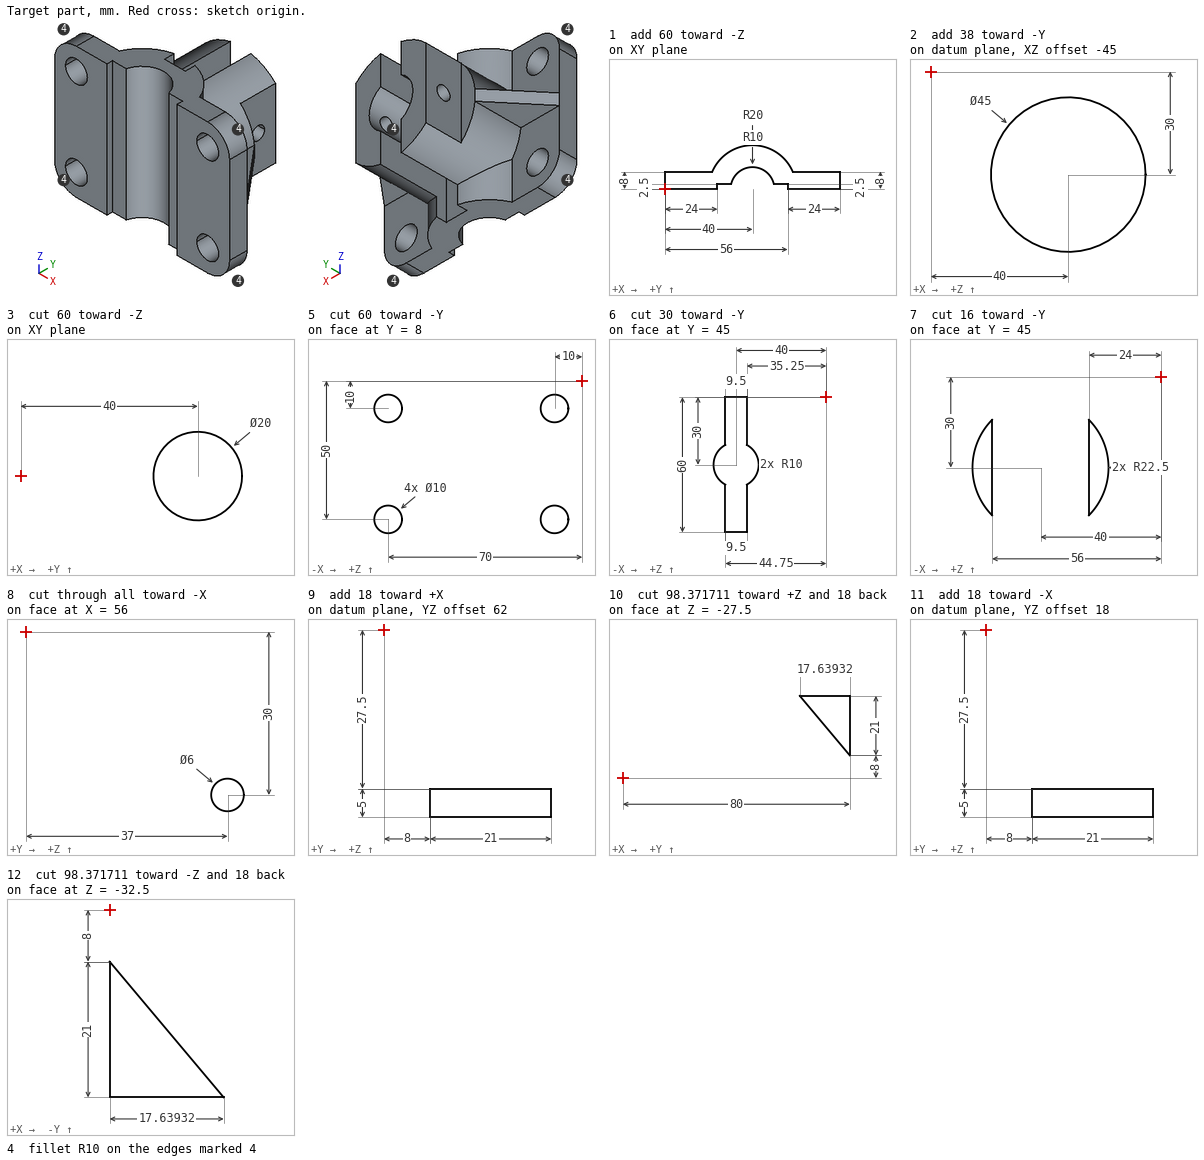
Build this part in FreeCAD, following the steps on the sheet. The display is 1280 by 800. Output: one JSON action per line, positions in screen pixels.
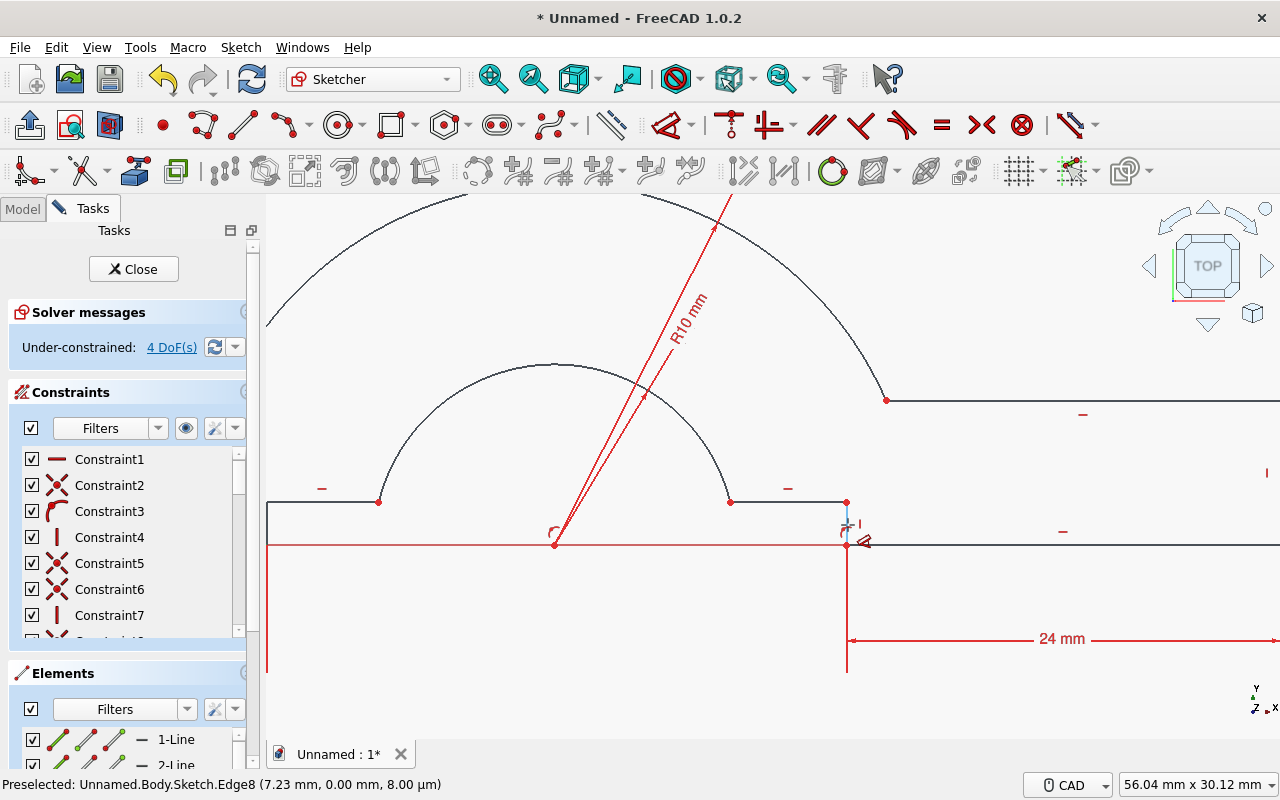
{"action": "left_click", "coordinate": [847, 524]}
{"action": "left_click", "coordinate": [881, 524]}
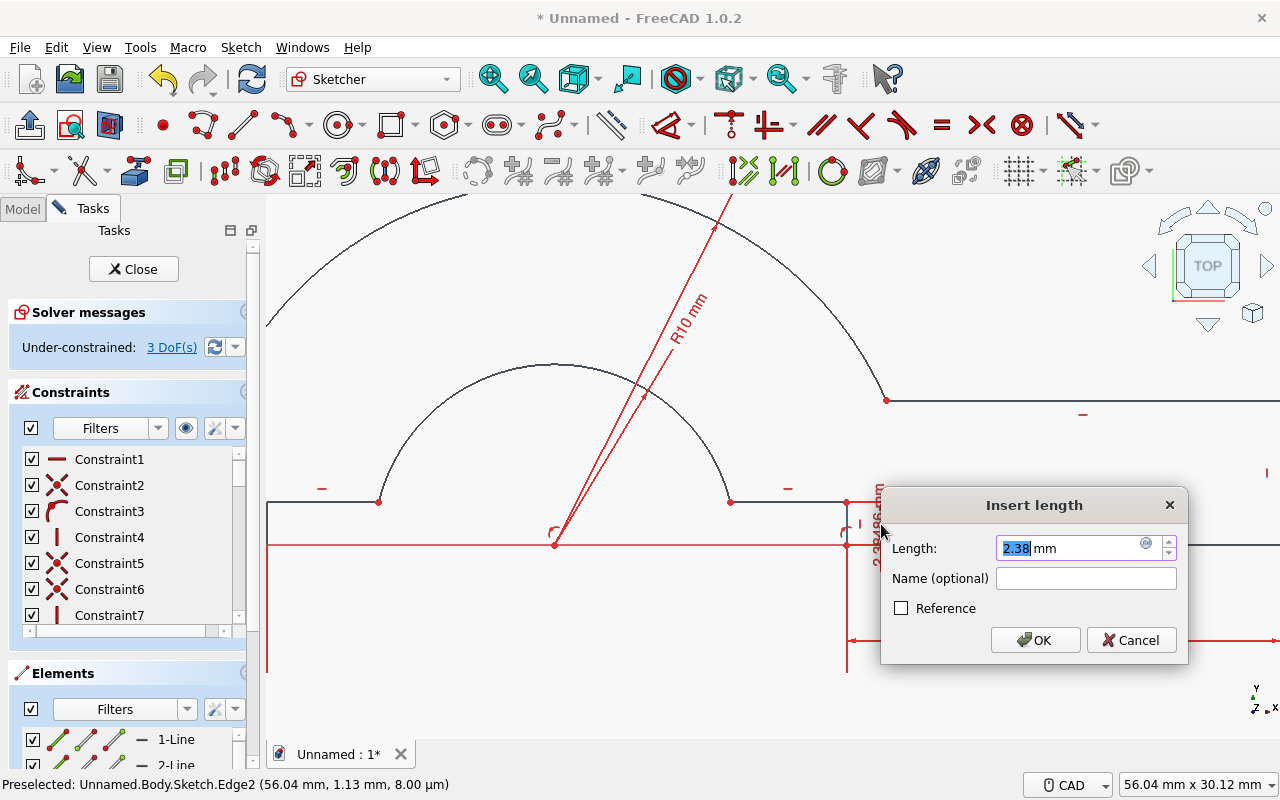
{"action": "type", "text": "2.5"}
{"action": "key", "text": "Return"}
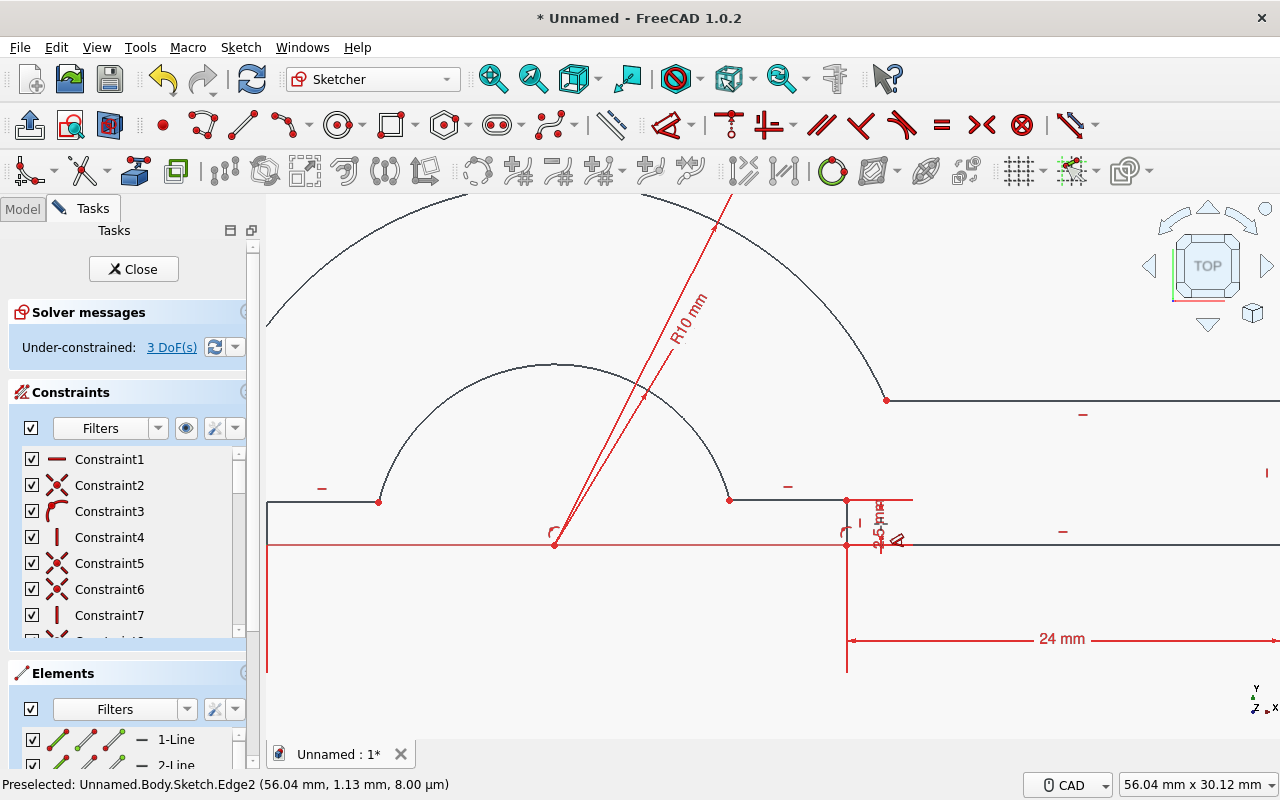
{"action": "scroll", "coordinate": [791, 526], "scroll_direction": "down", "scroll_amount": 5}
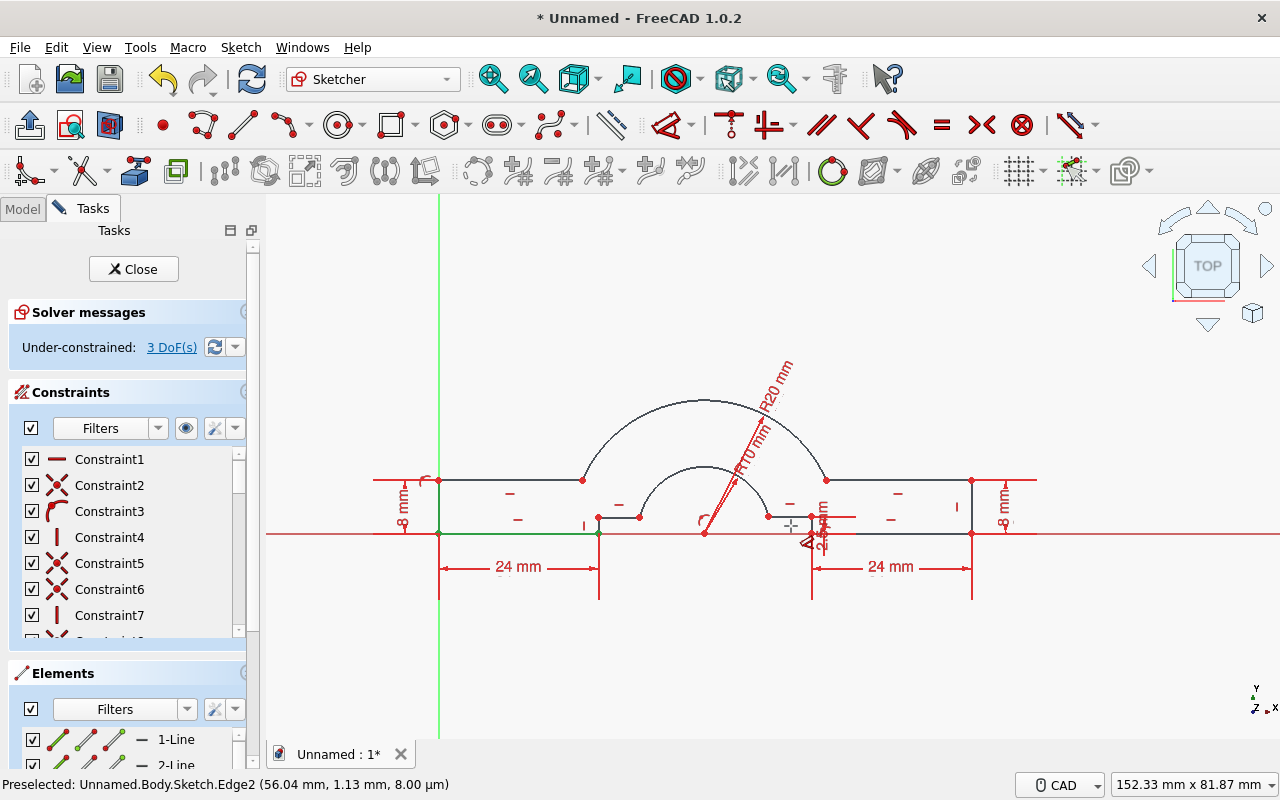
{"action": "scroll", "coordinate": [599, 529], "scroll_direction": "up", "scroll_amount": 6}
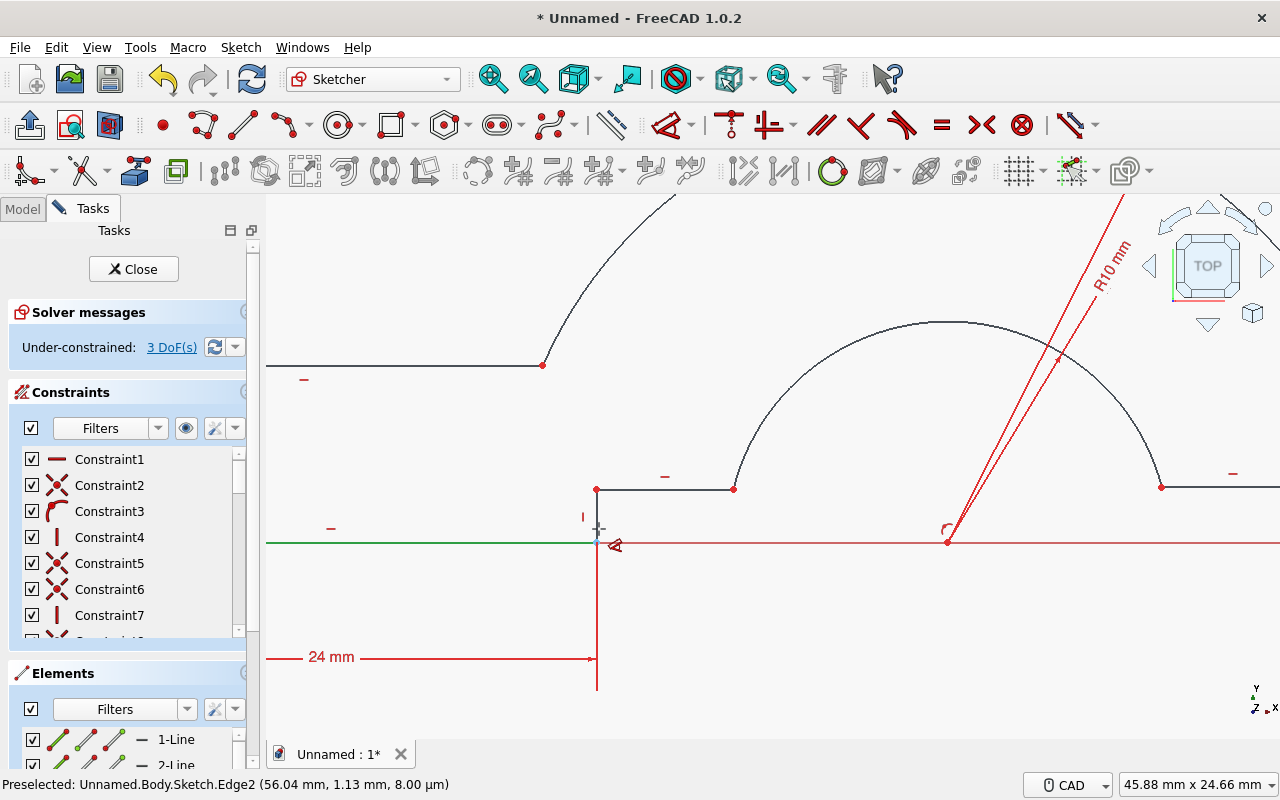
{"action": "left_click", "coordinate": [597, 527]}
{"action": "left_click", "coordinate": [563, 516]}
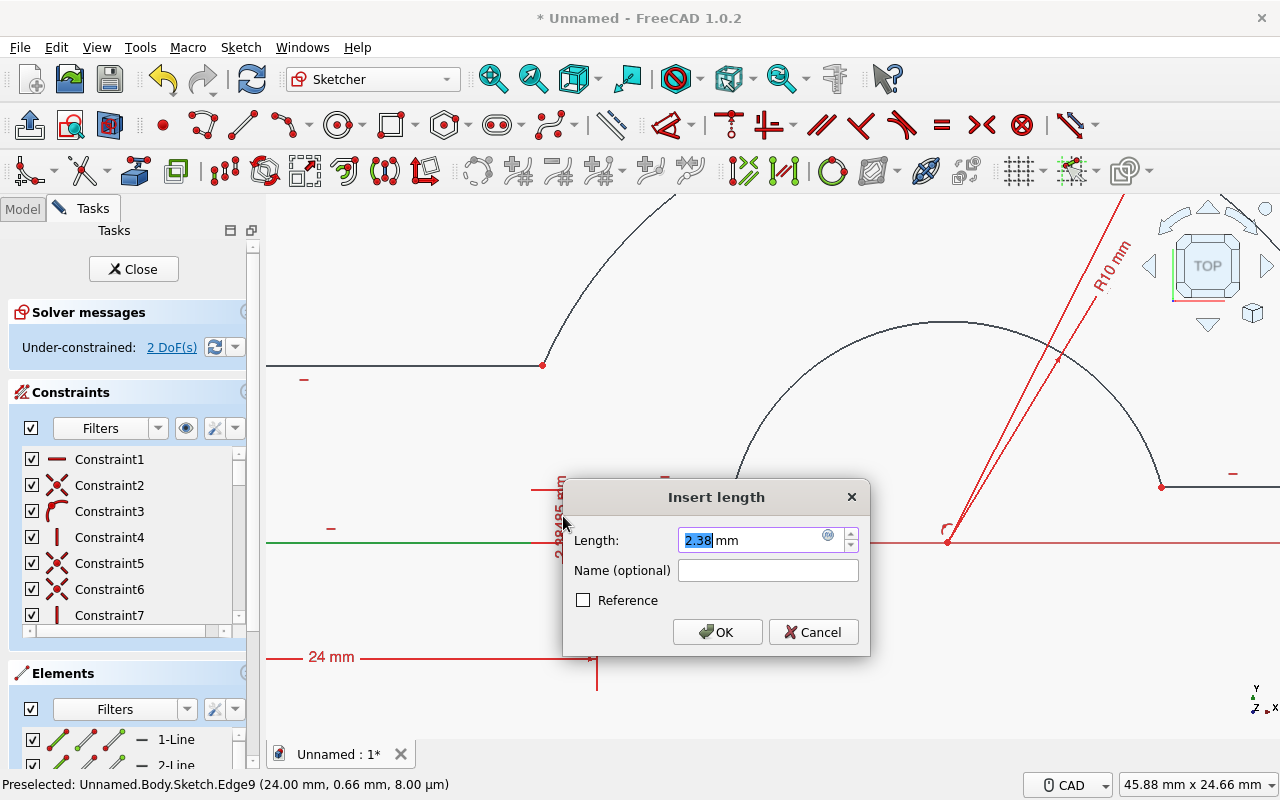
{"action": "type", "text": "2.5"}
{"action": "key", "text": "Return"}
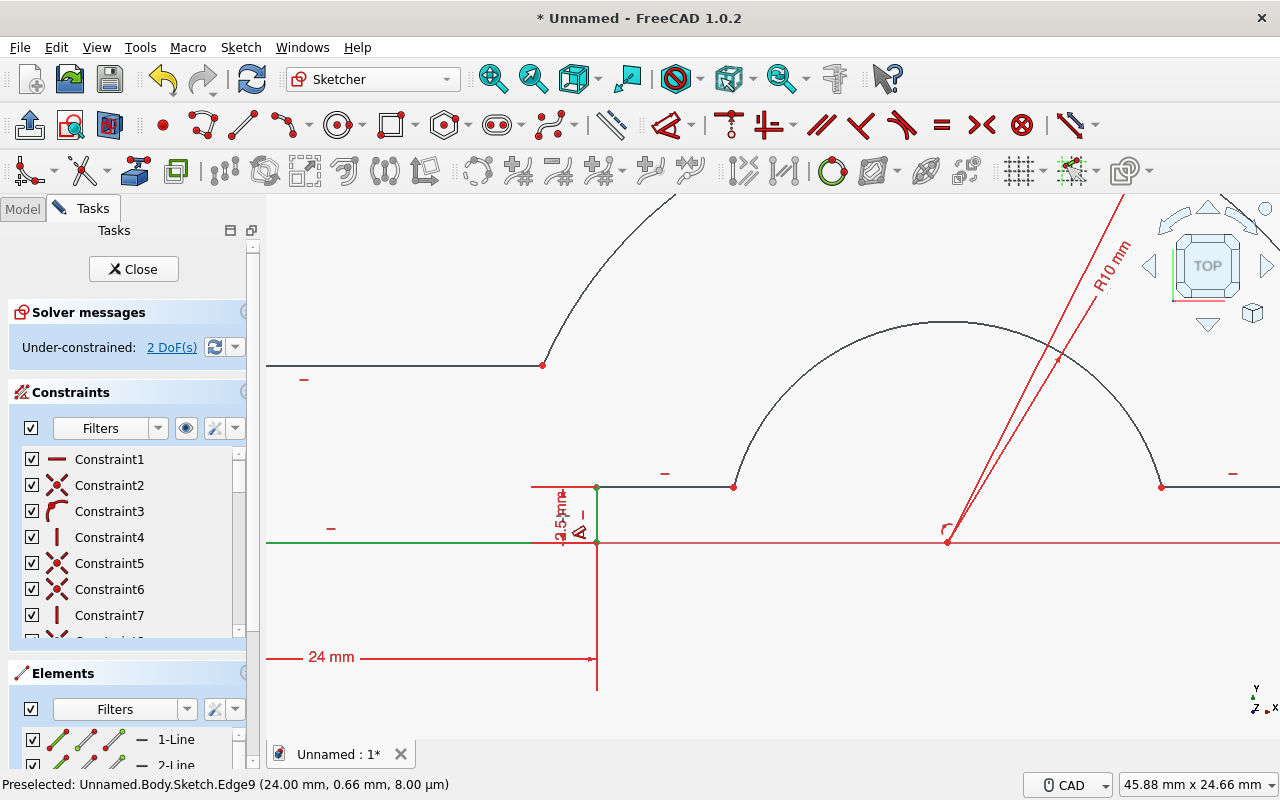
{"action": "scroll", "coordinate": [599, 529], "scroll_direction": "down", "scroll_amount": 6}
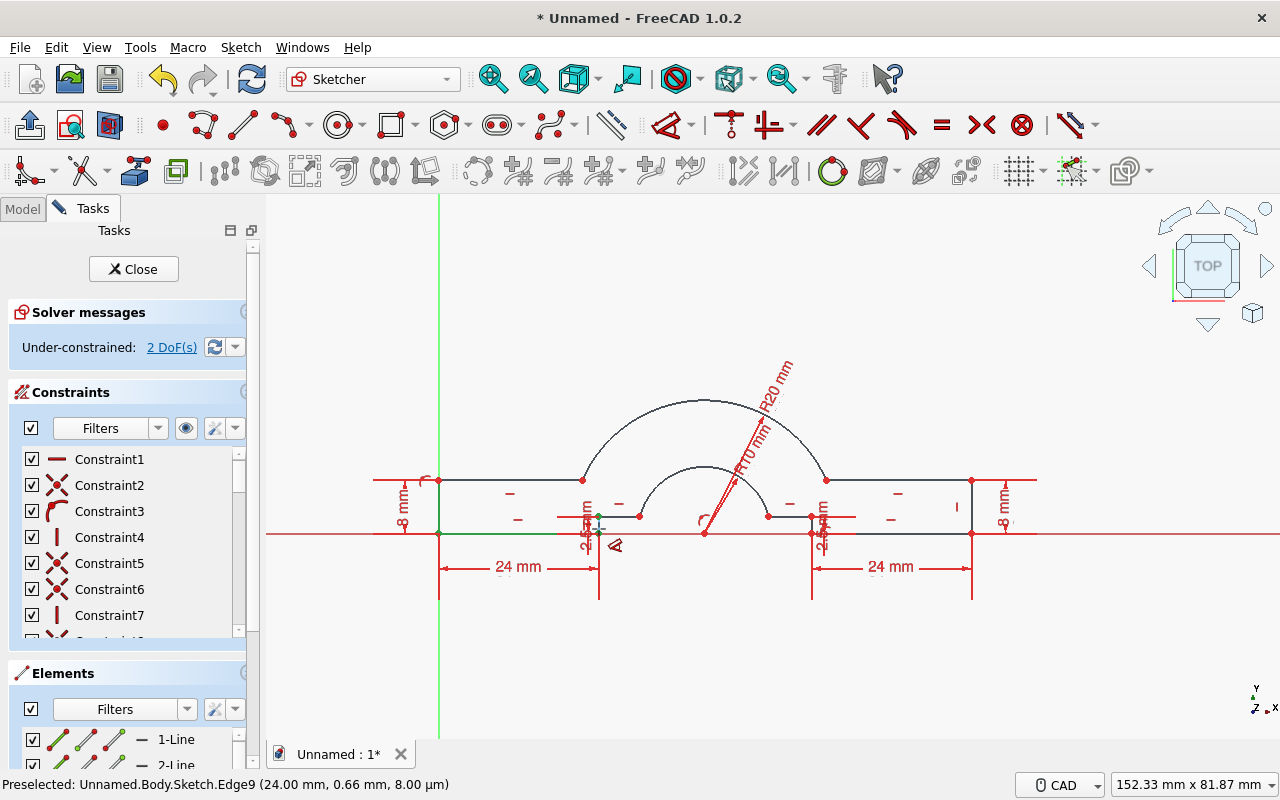
{"action": "left_click", "coordinate": [812, 517]}
{"action": "left_click", "coordinate": [625, 568]}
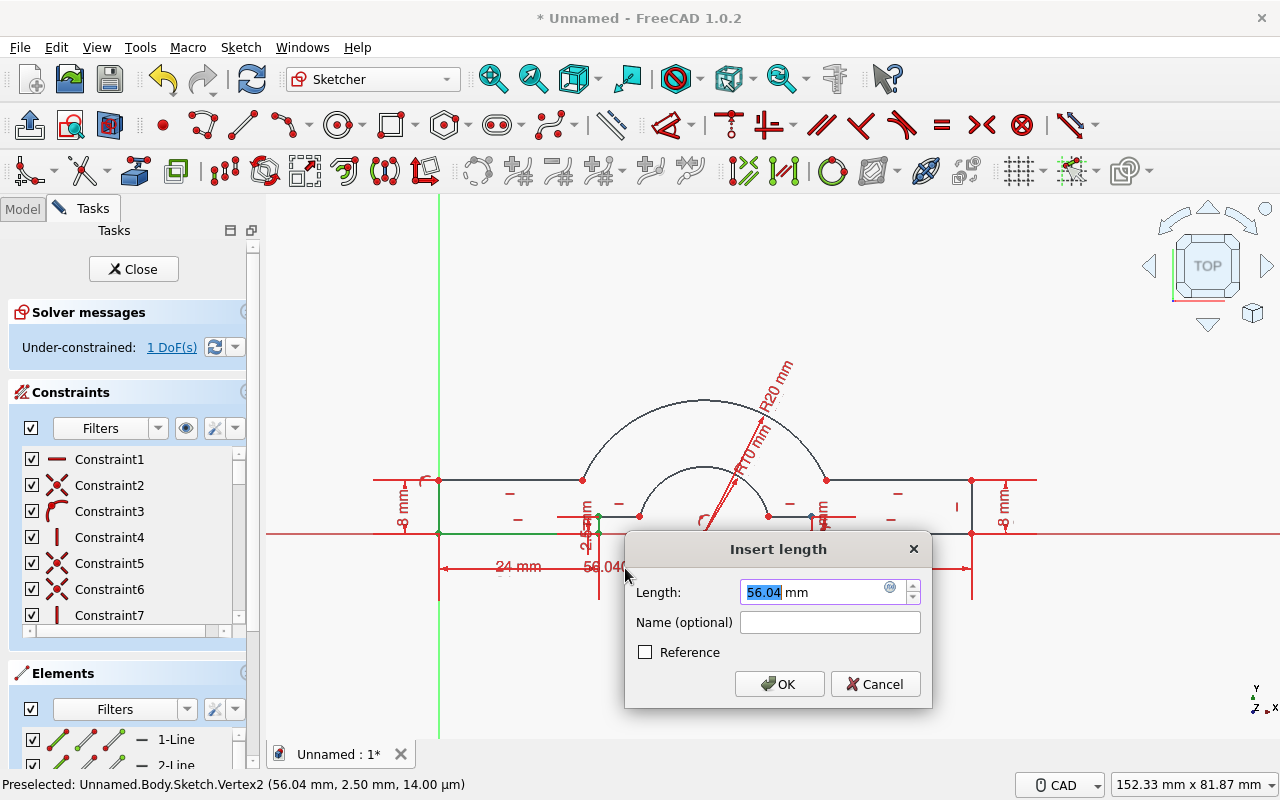
{"action": "type", "text": "56"}
{"action": "key", "text": "Return"}